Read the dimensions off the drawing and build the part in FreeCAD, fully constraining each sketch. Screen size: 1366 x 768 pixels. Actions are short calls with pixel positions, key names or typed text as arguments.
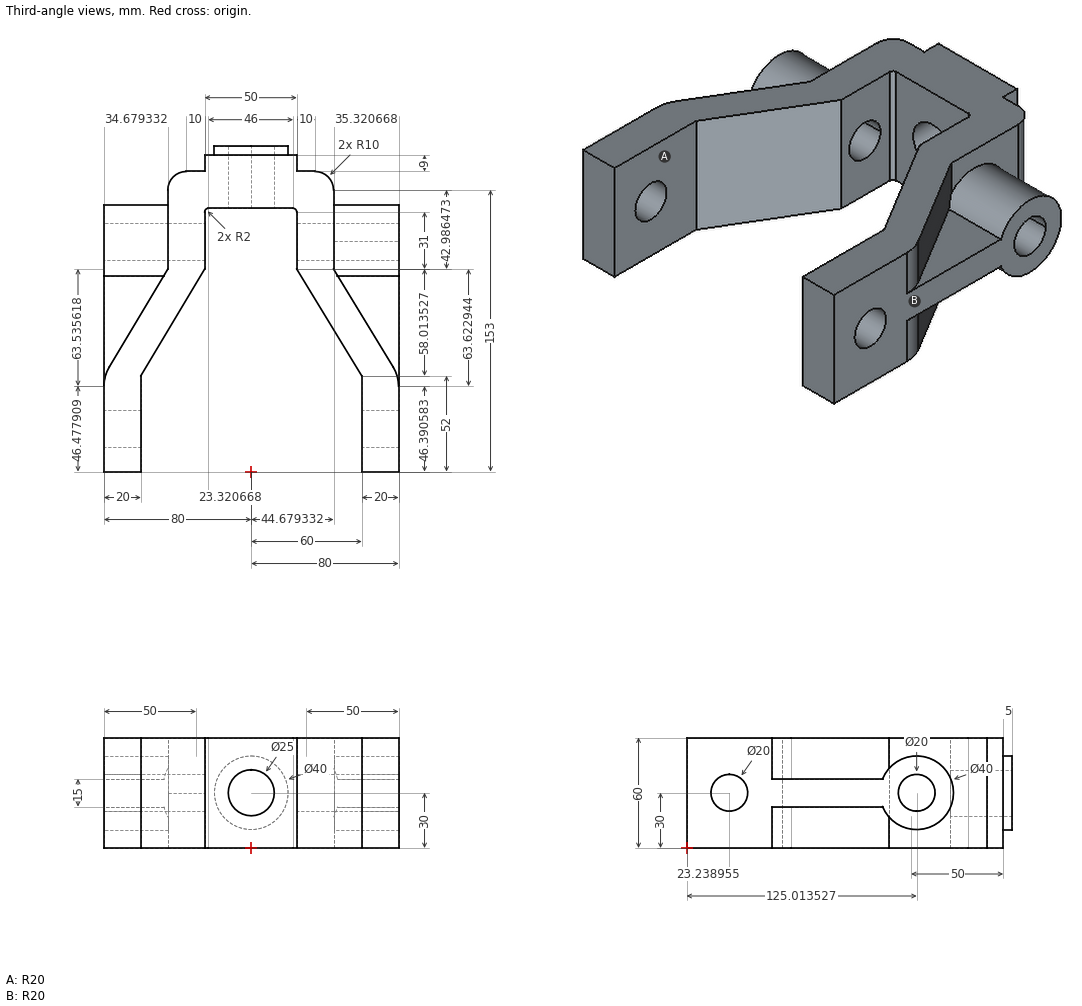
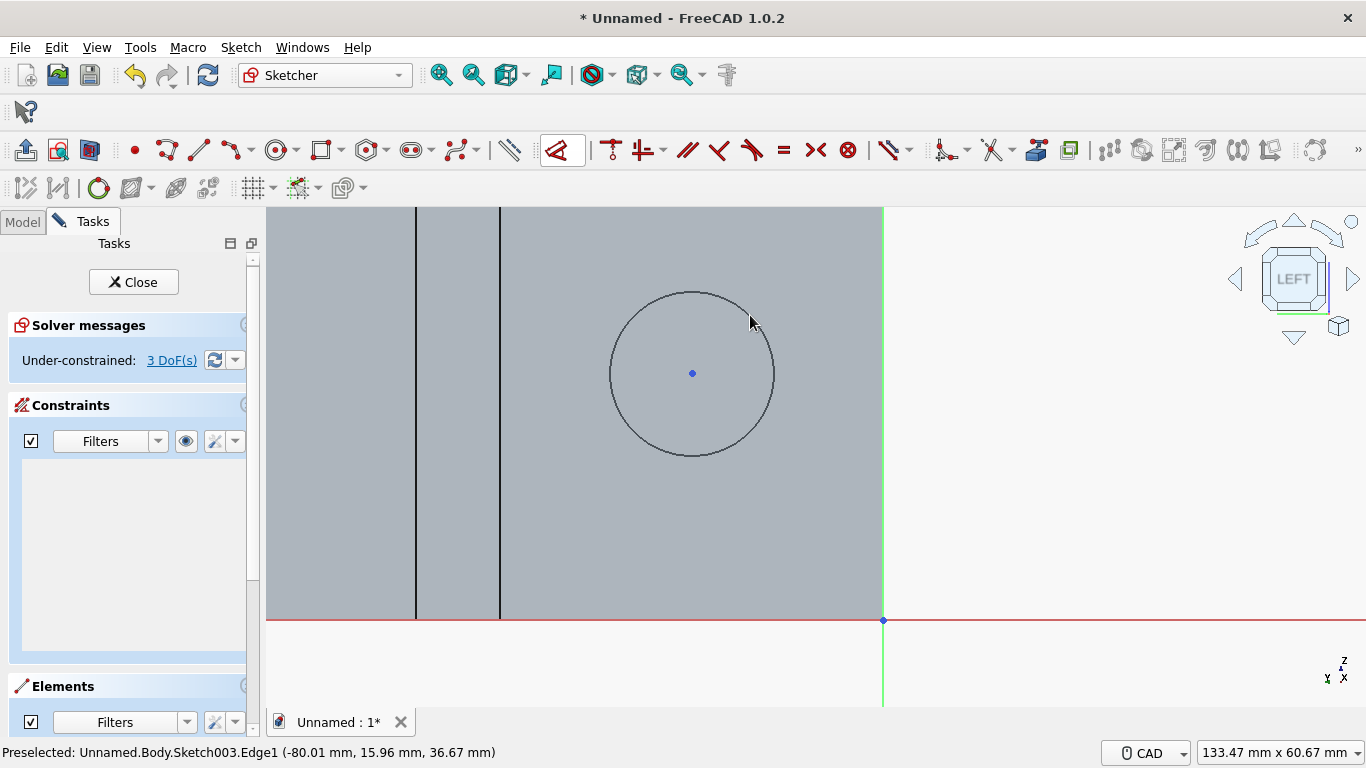
click(750, 316)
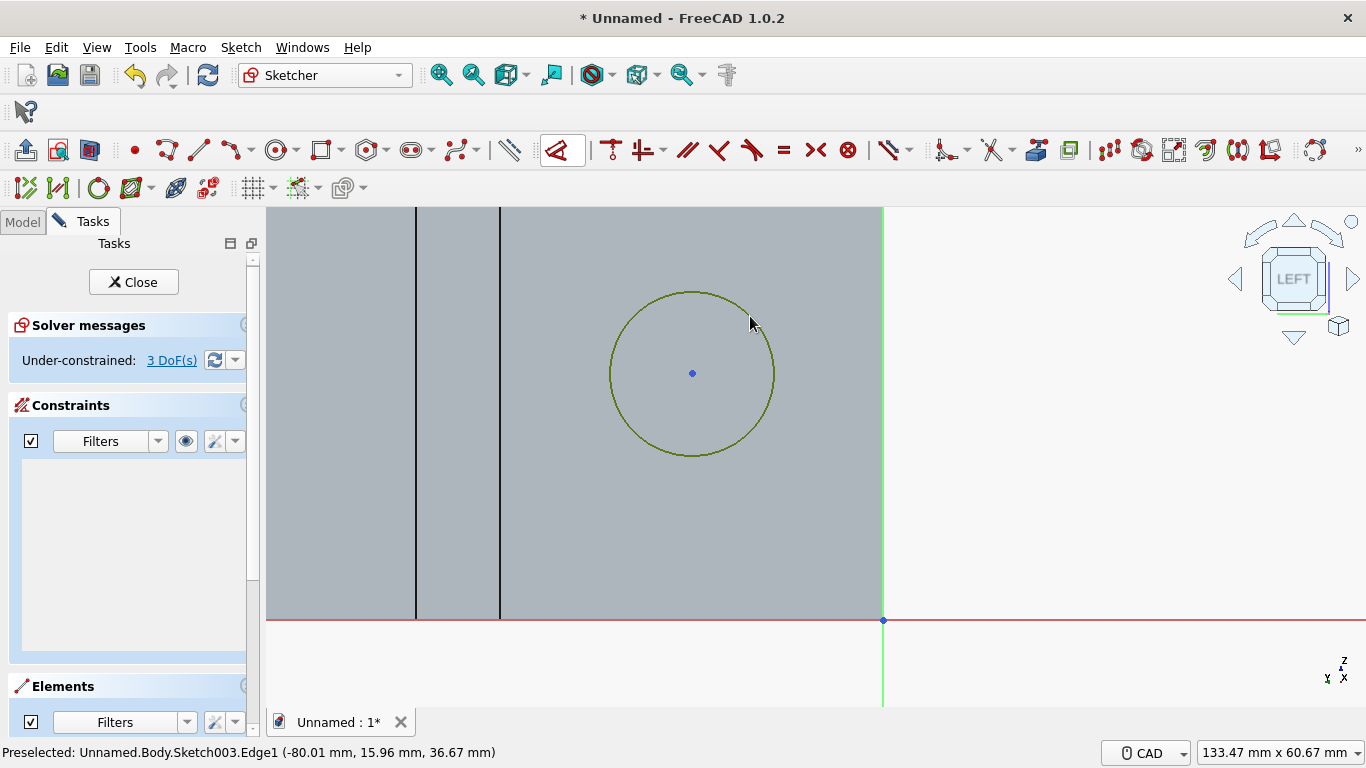
click(580, 150)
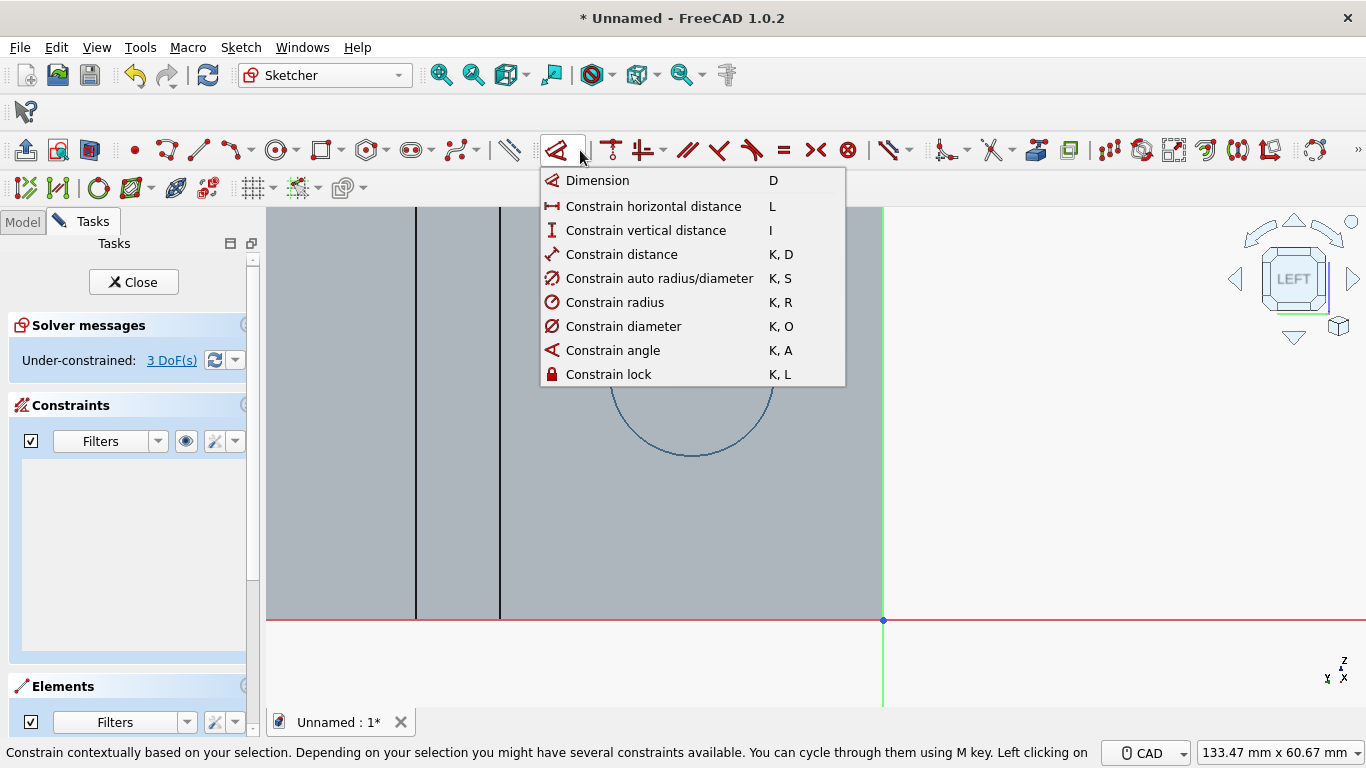
click(693, 326)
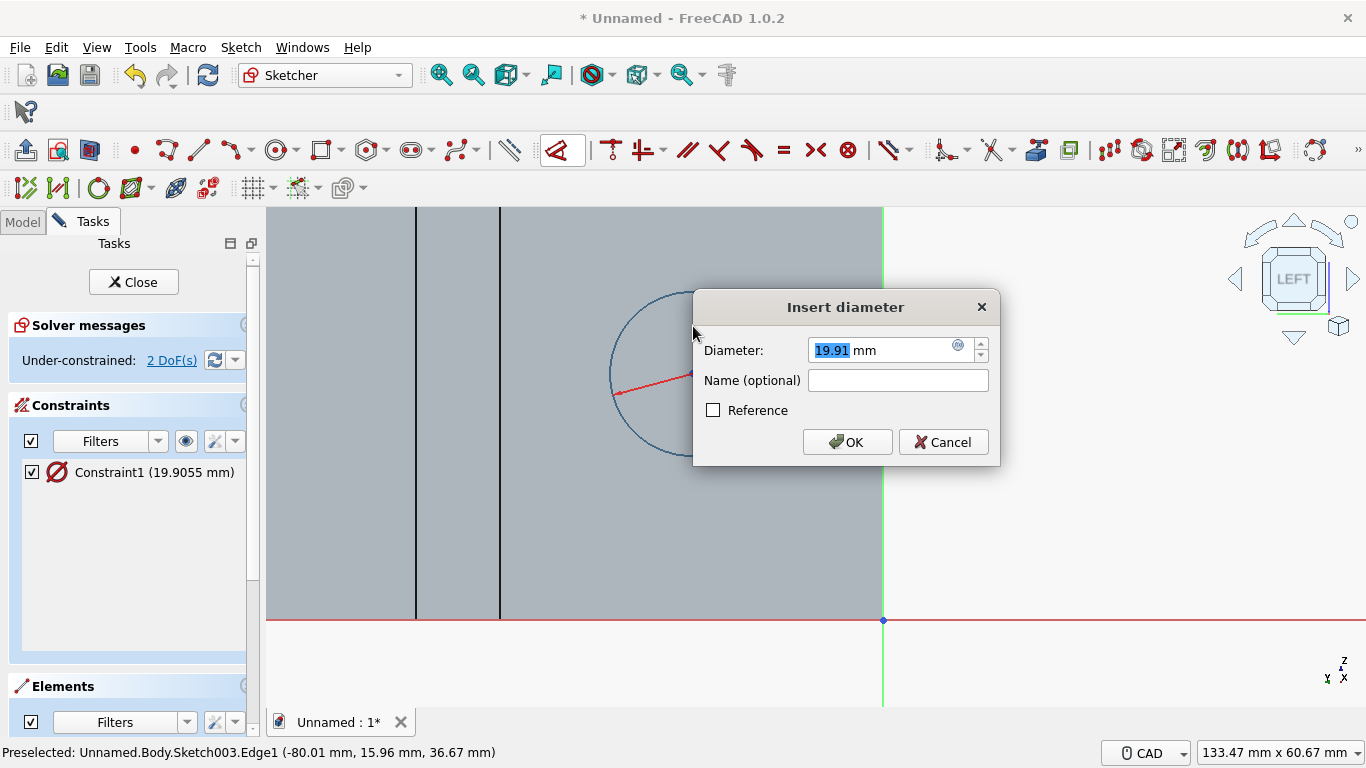
text(20)
key(Return)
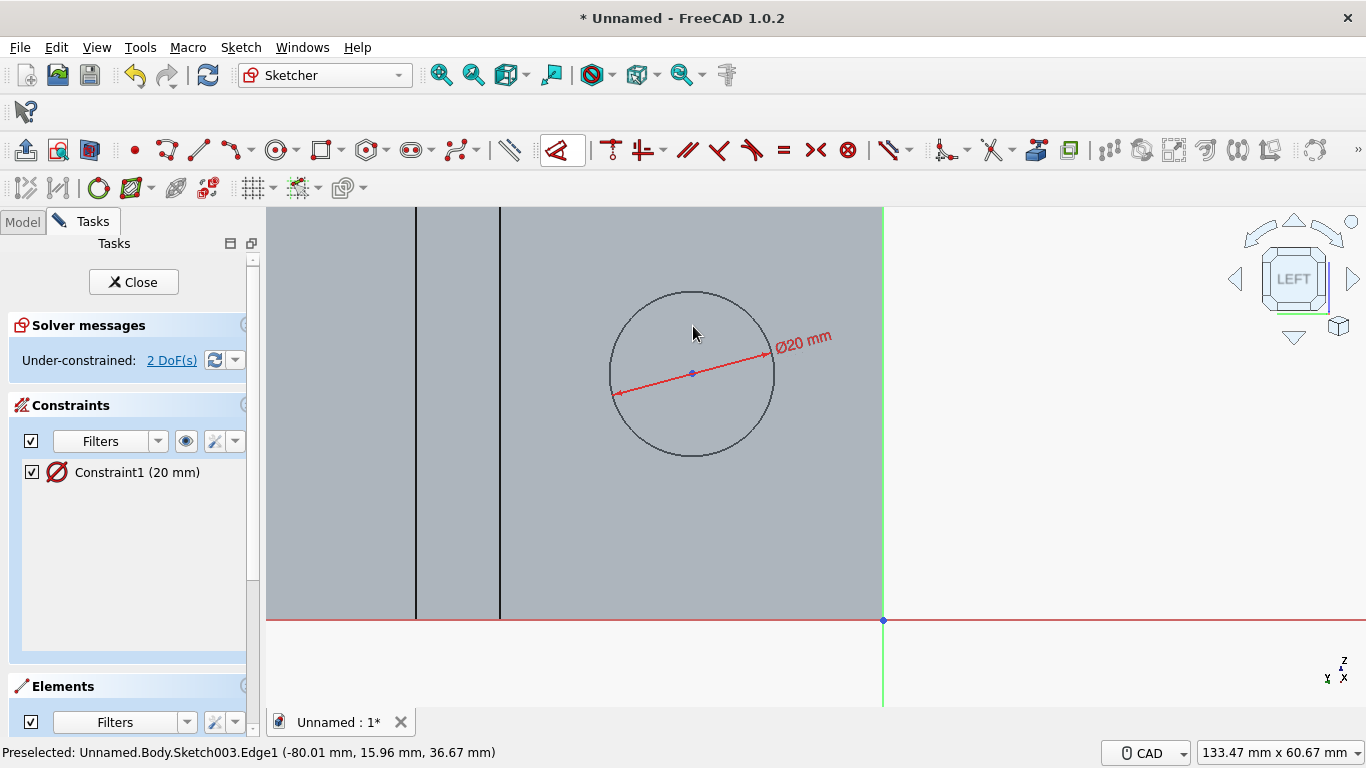
click(692, 374)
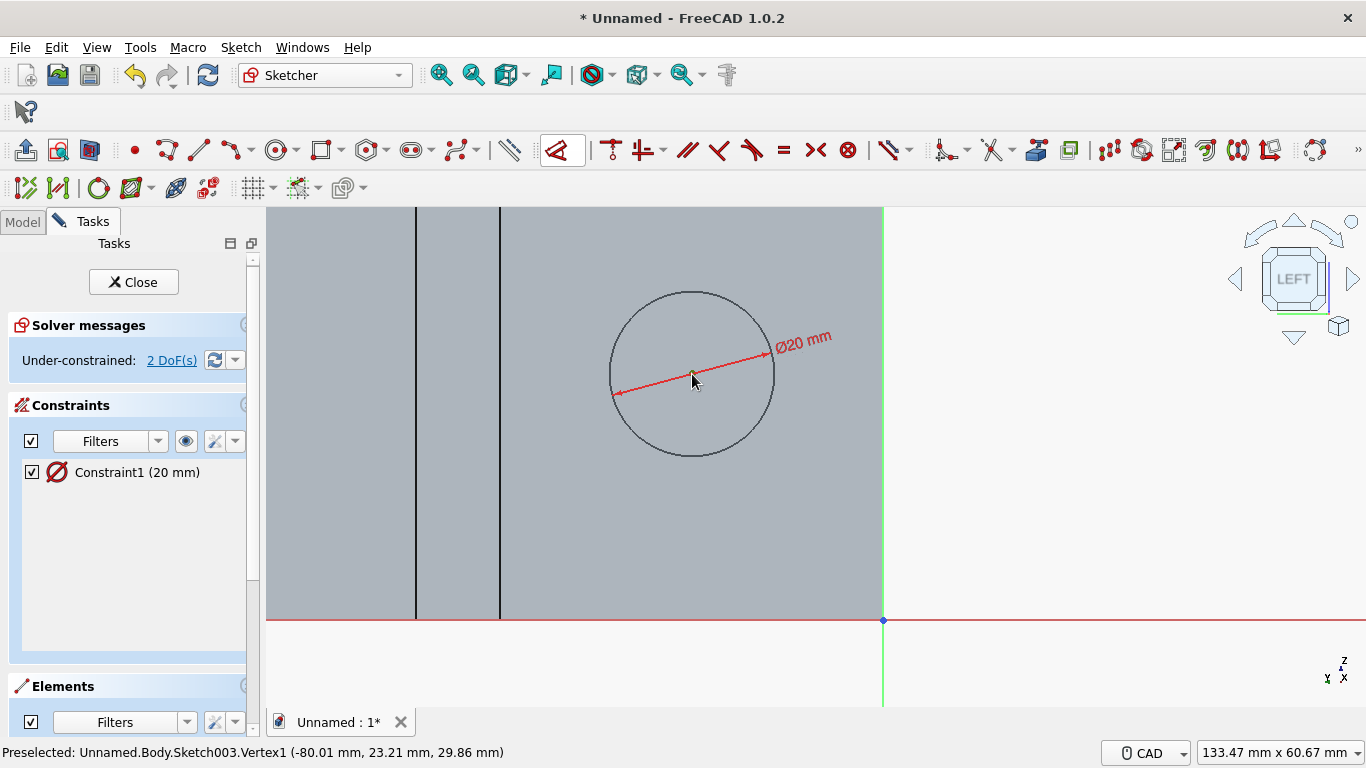
key(i)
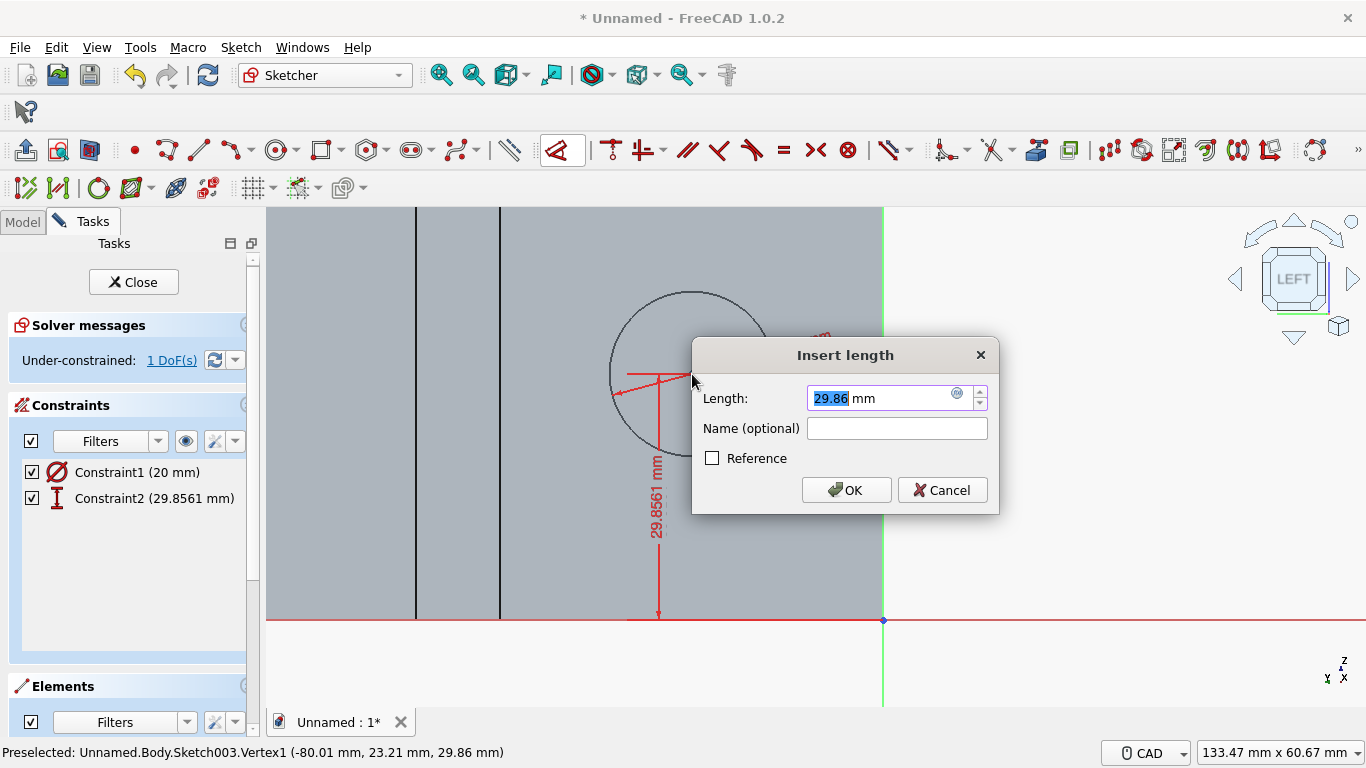
text(30)
key(Return)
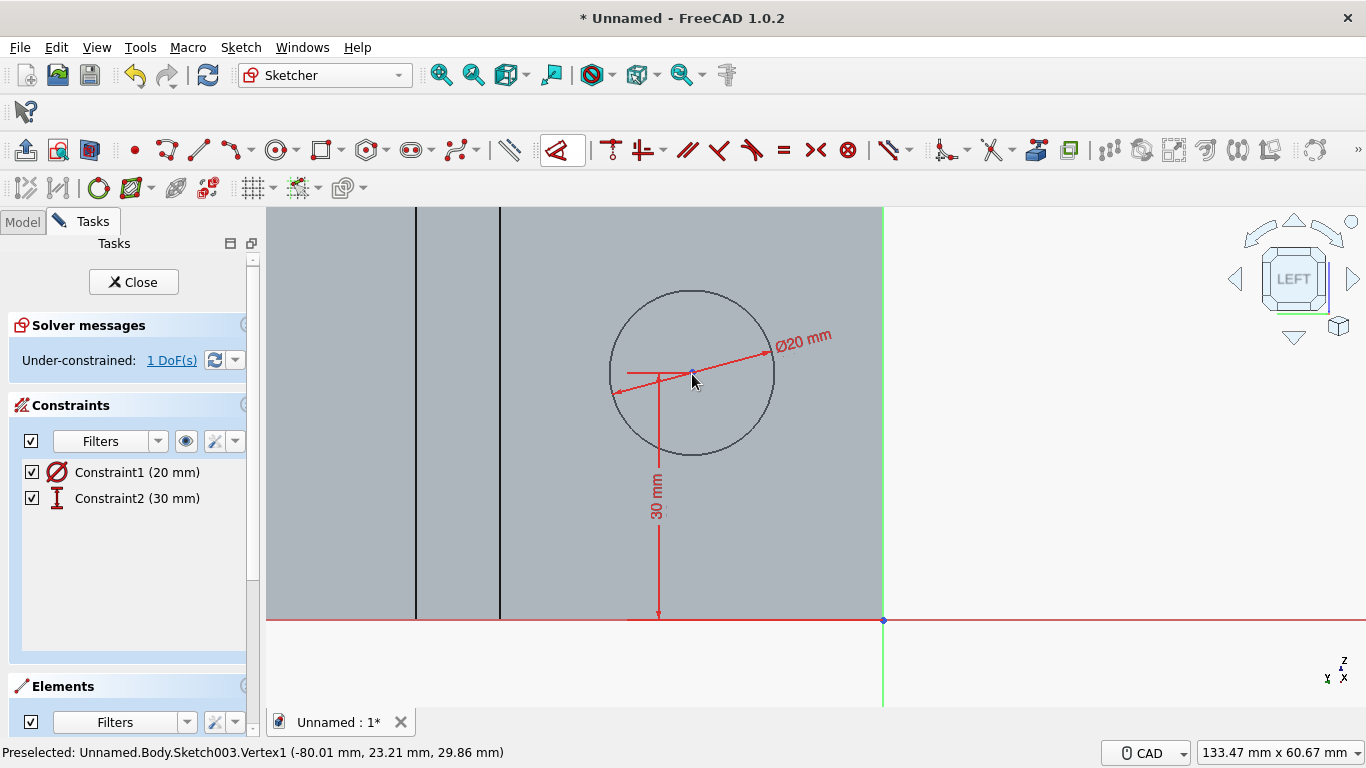
click(692, 373)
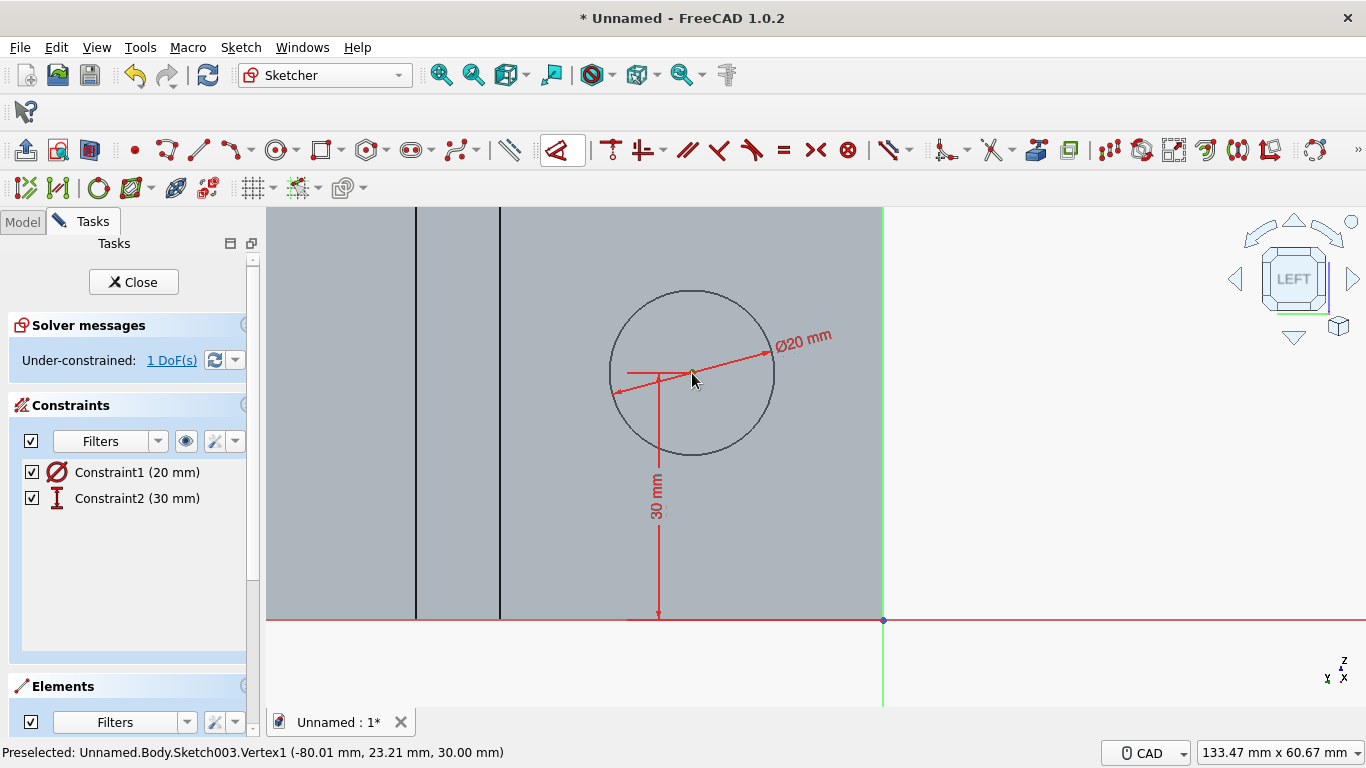
click(580, 150)